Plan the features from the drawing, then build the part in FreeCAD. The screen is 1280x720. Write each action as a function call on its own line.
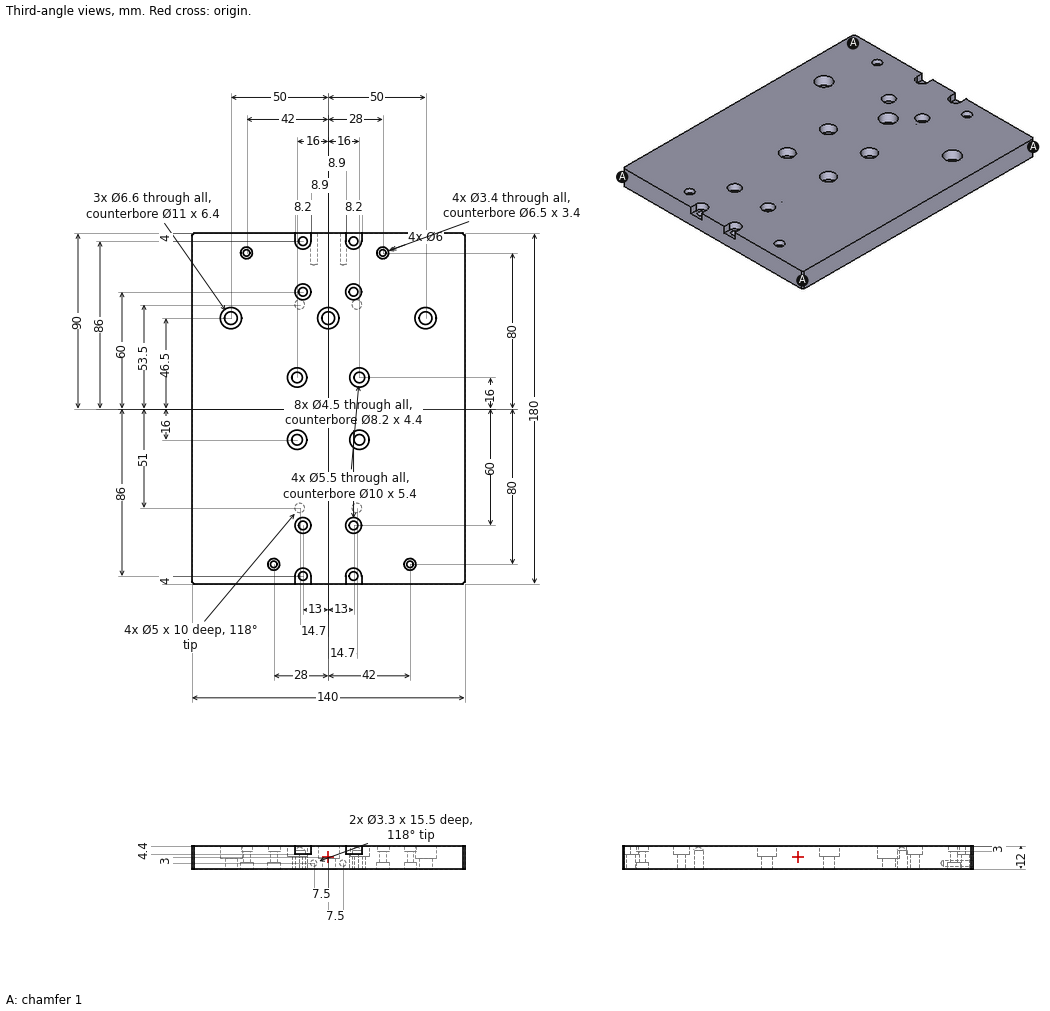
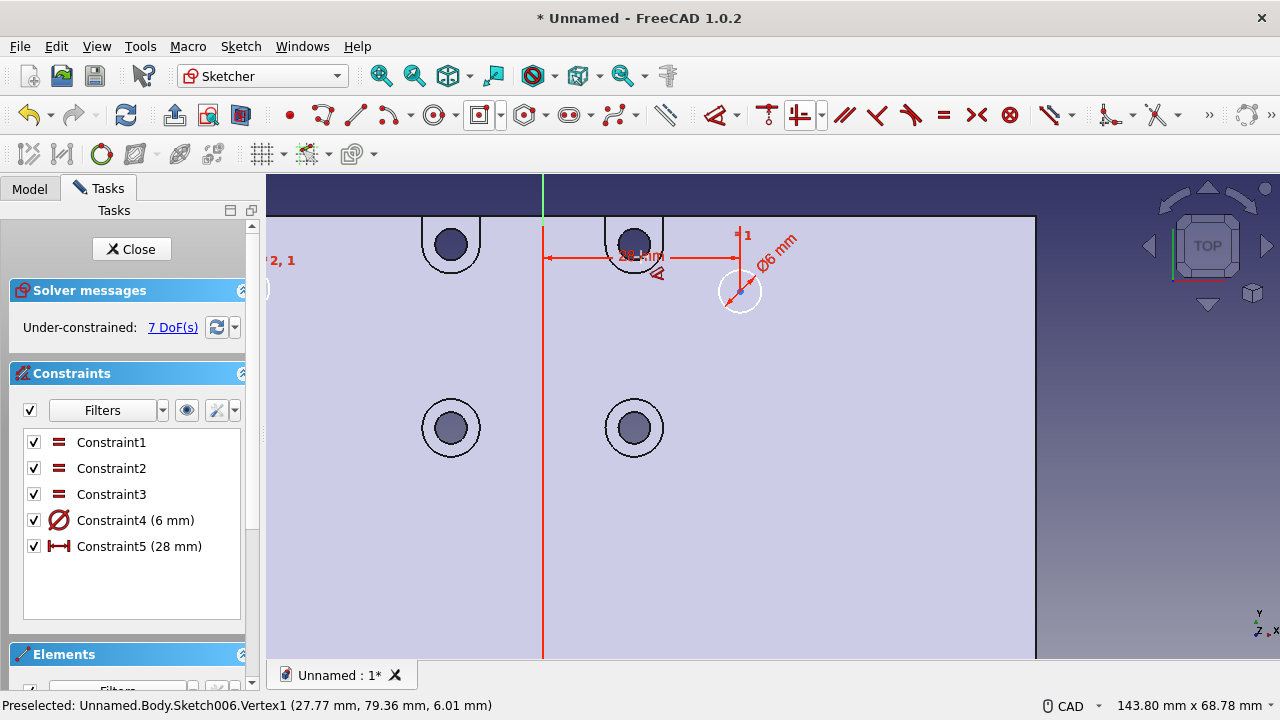
click(740, 291)
click(774, 461)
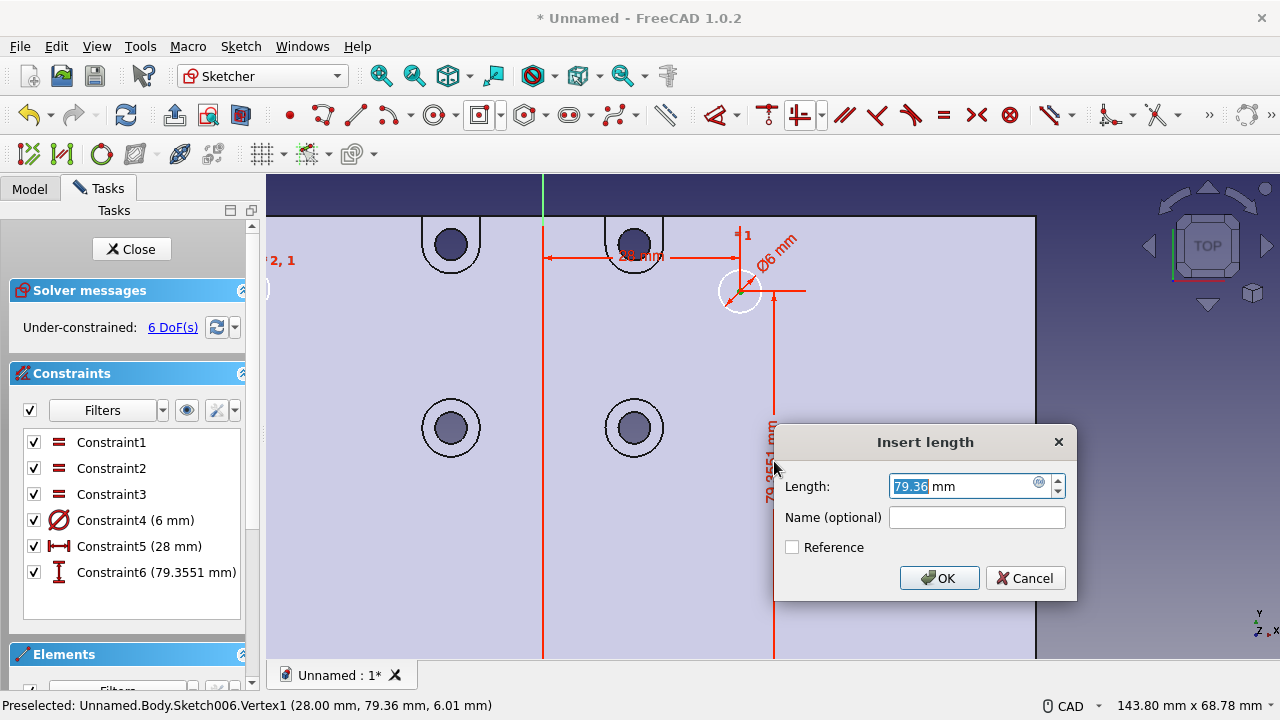
text(80)
key(Return)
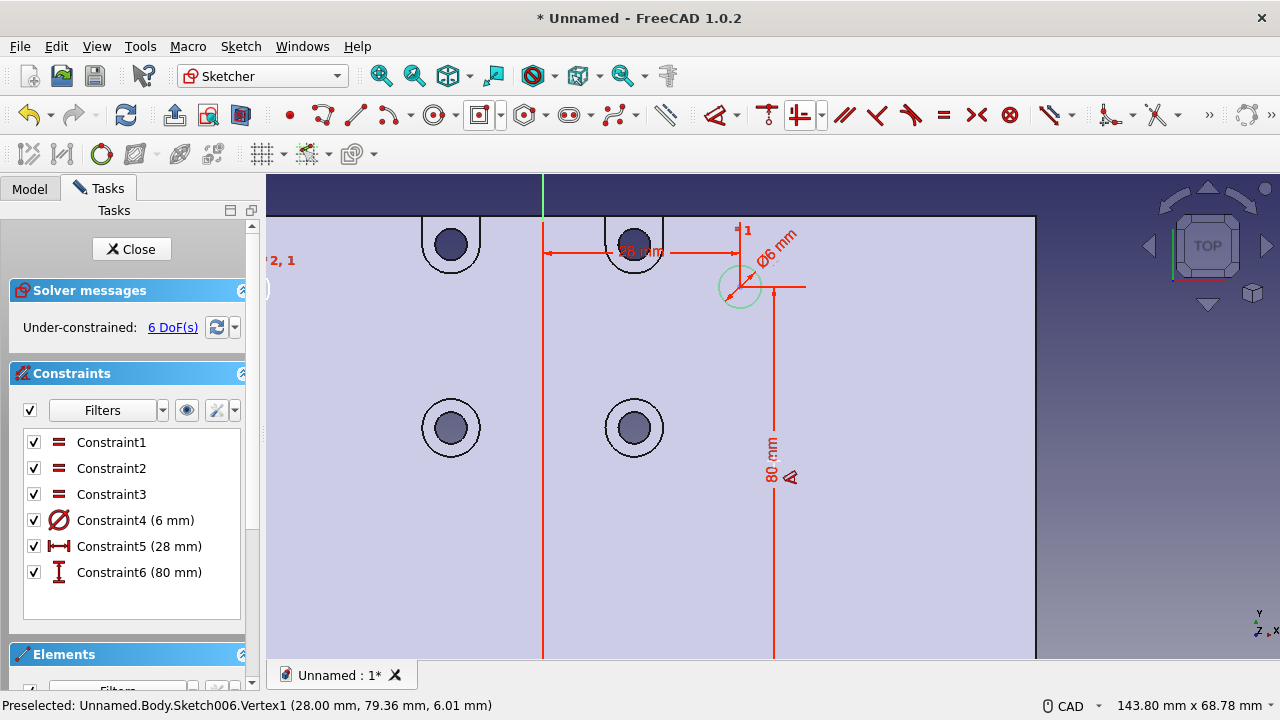
scroll(757, 274, down, 7)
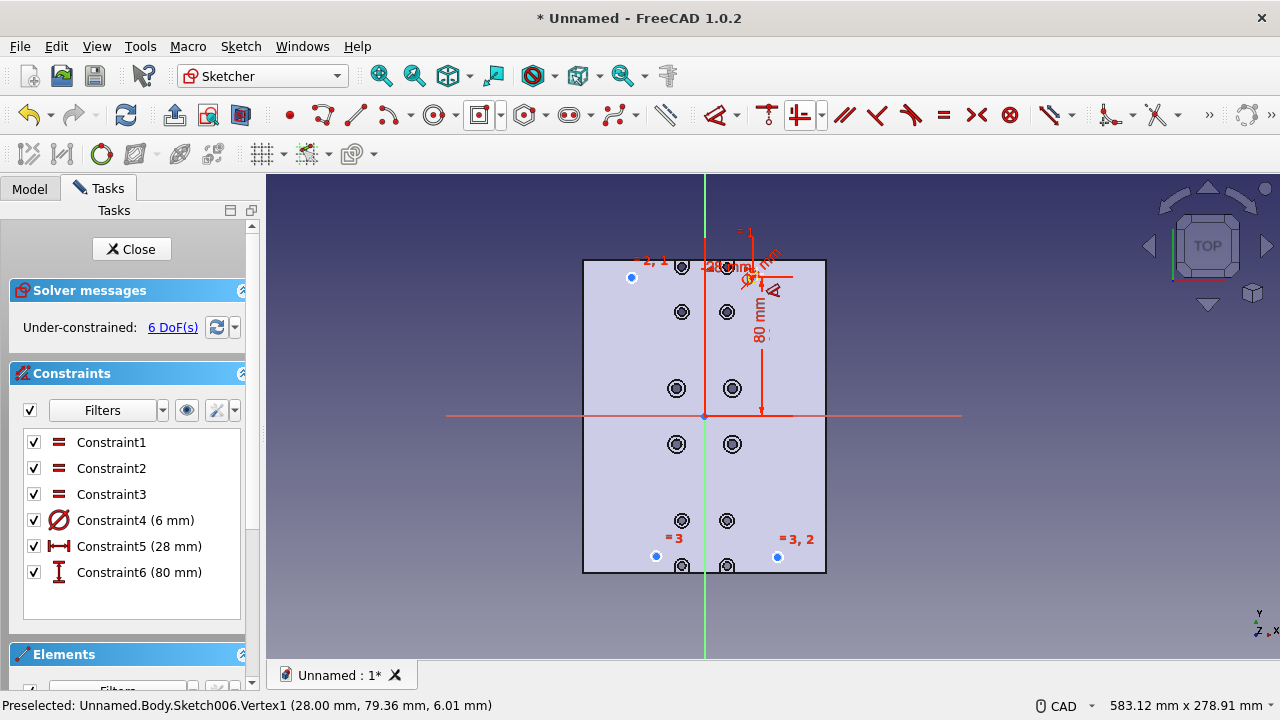
click(632, 278)
click(668, 244)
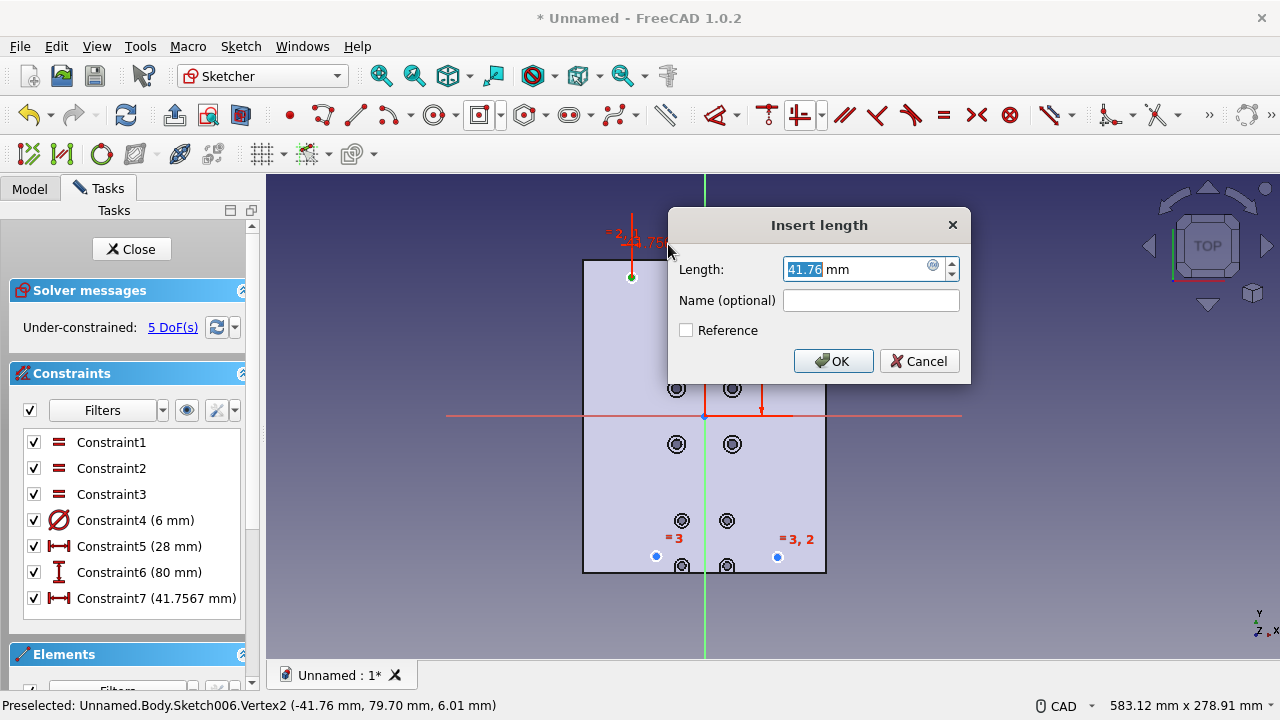
text(42)
key(Return)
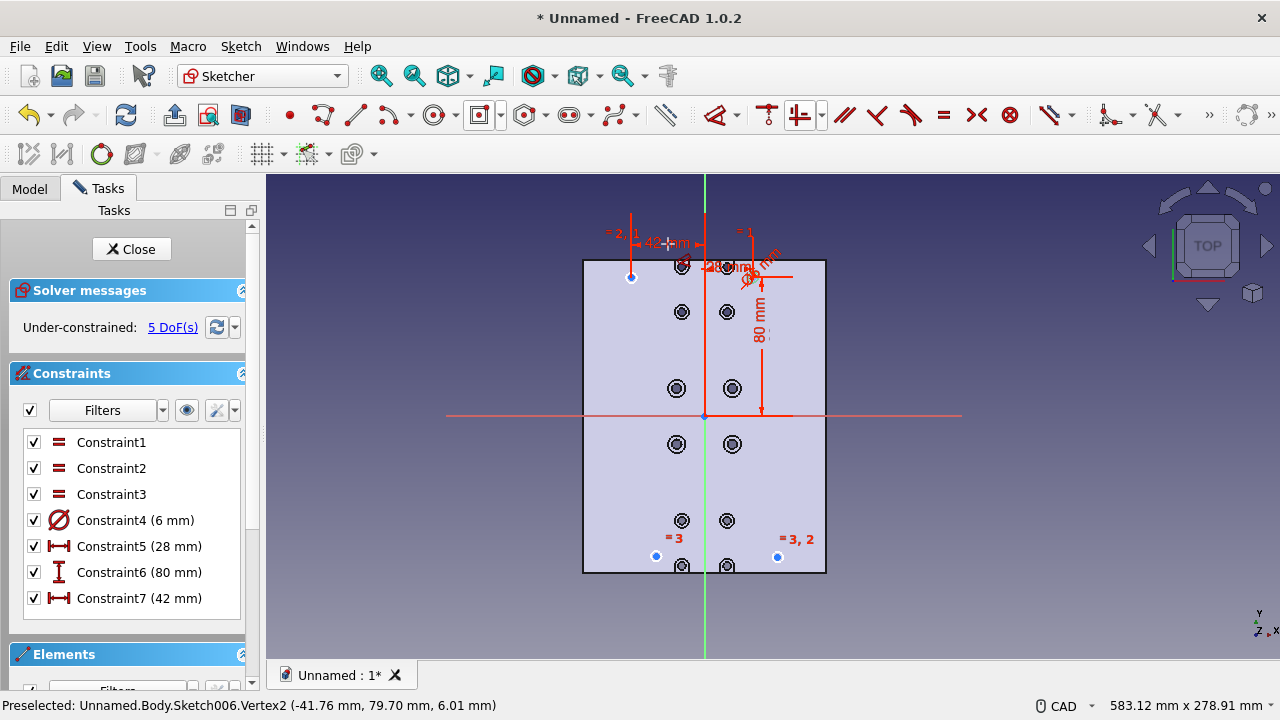
click(631, 278)
click(597, 347)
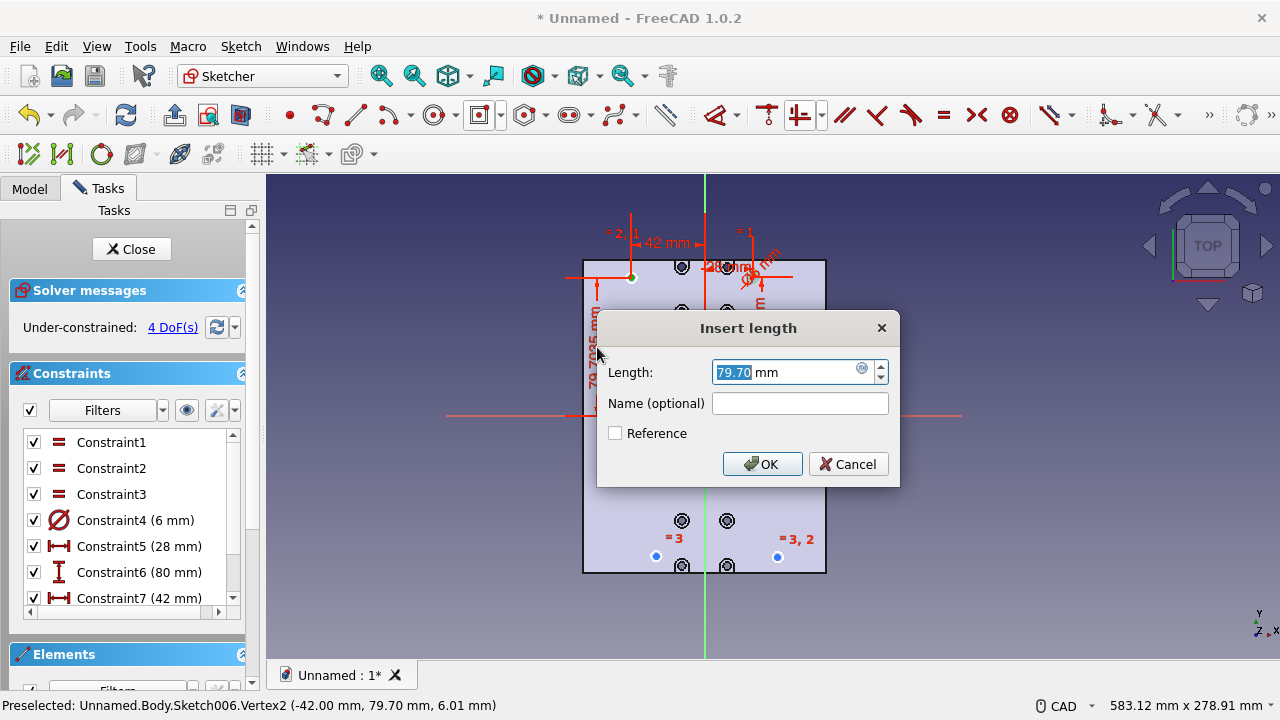
text(80)
key(Return)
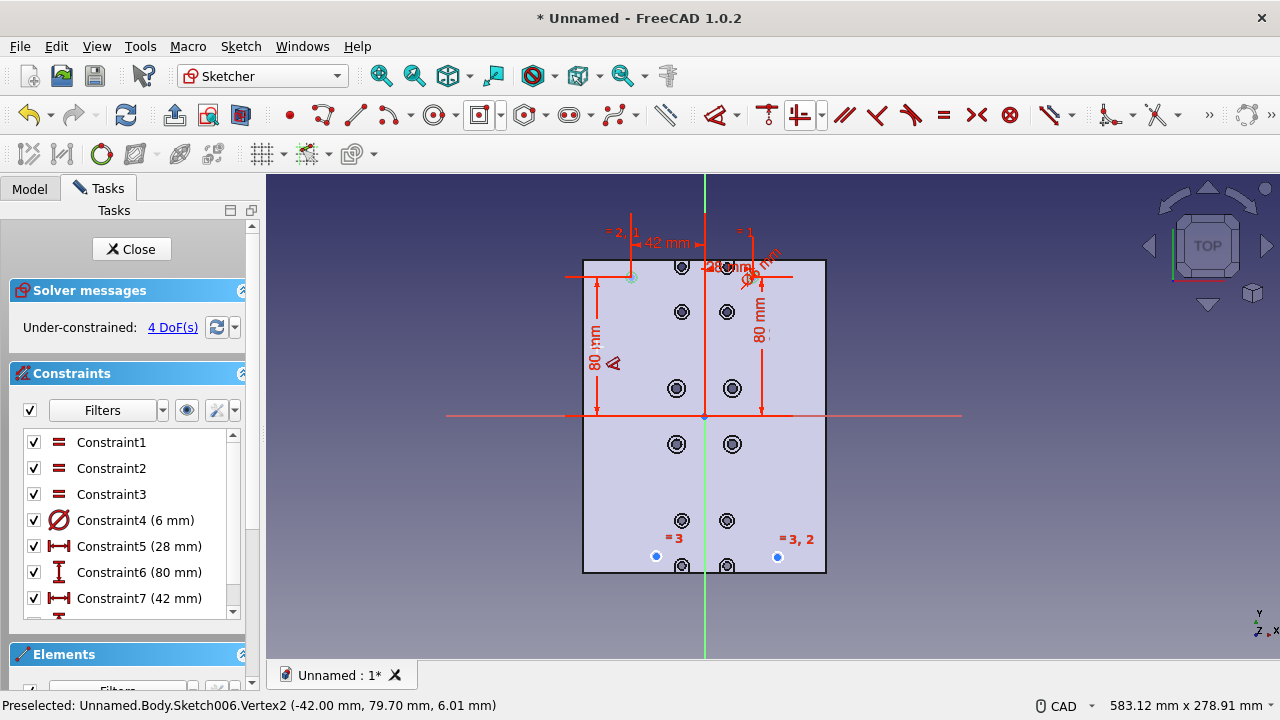
click(778, 557)
click(741, 591)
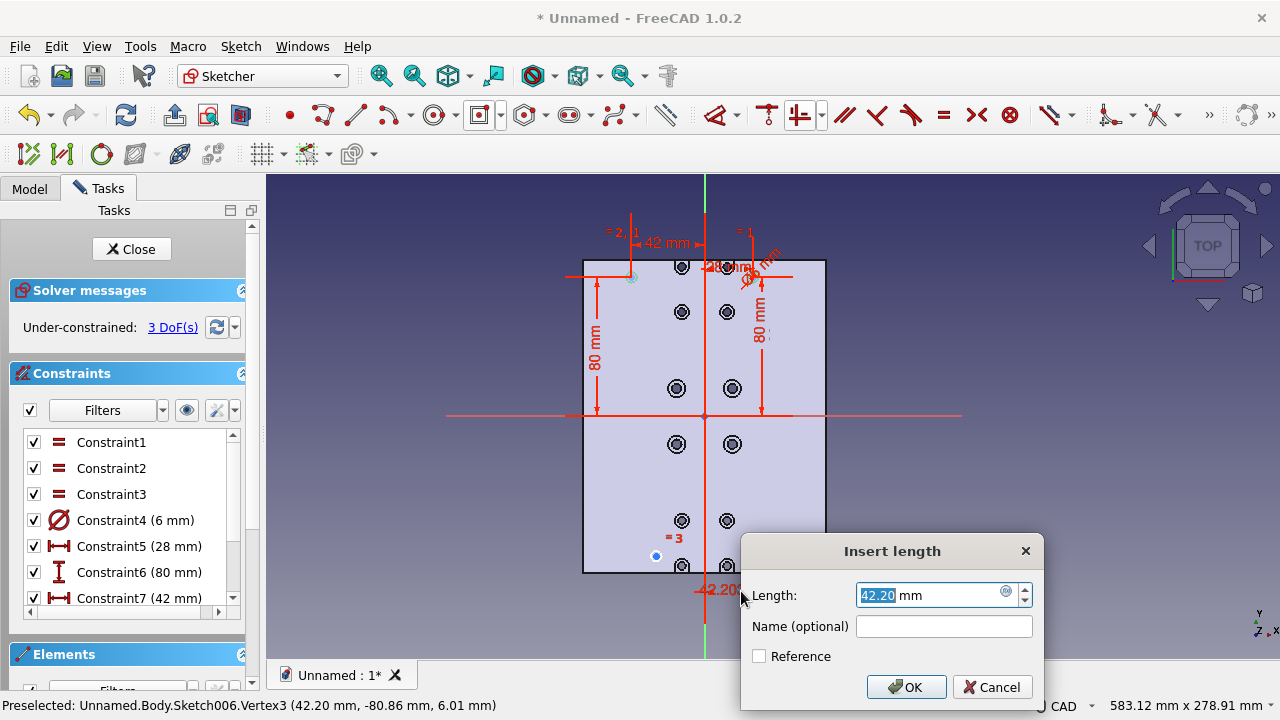
text(42)
key(Return)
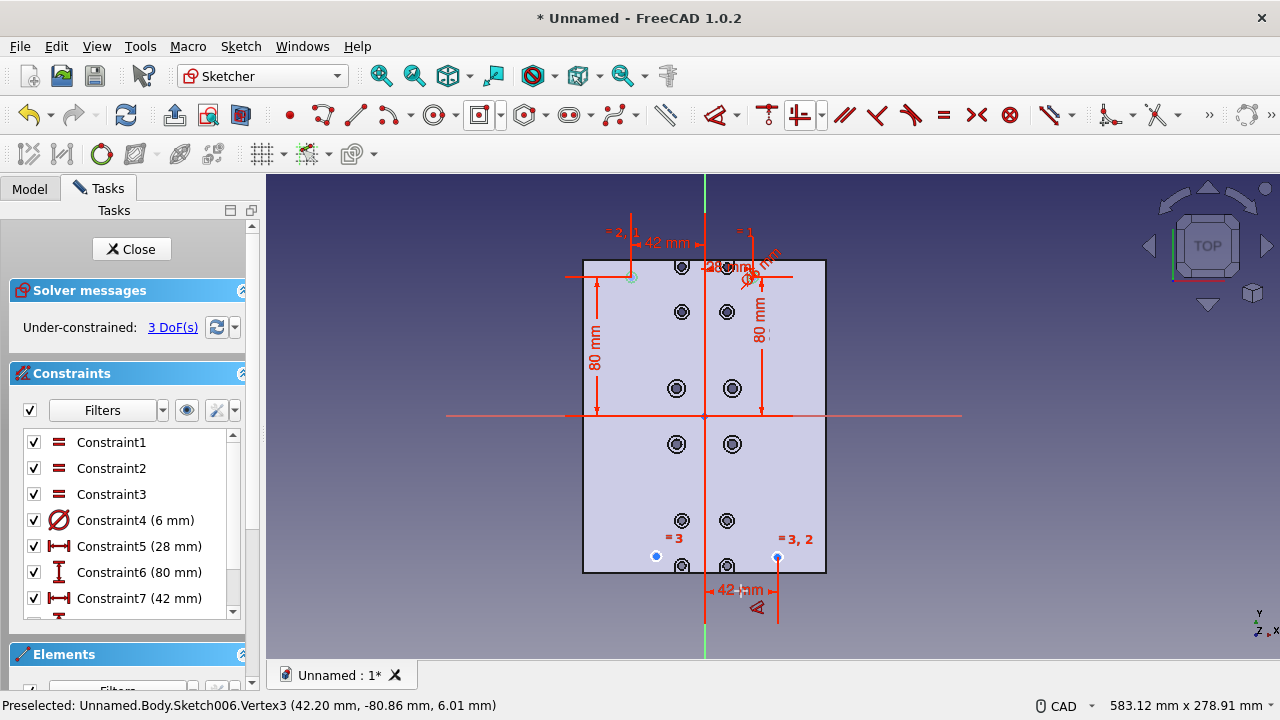
click(778, 557)
click(812, 487)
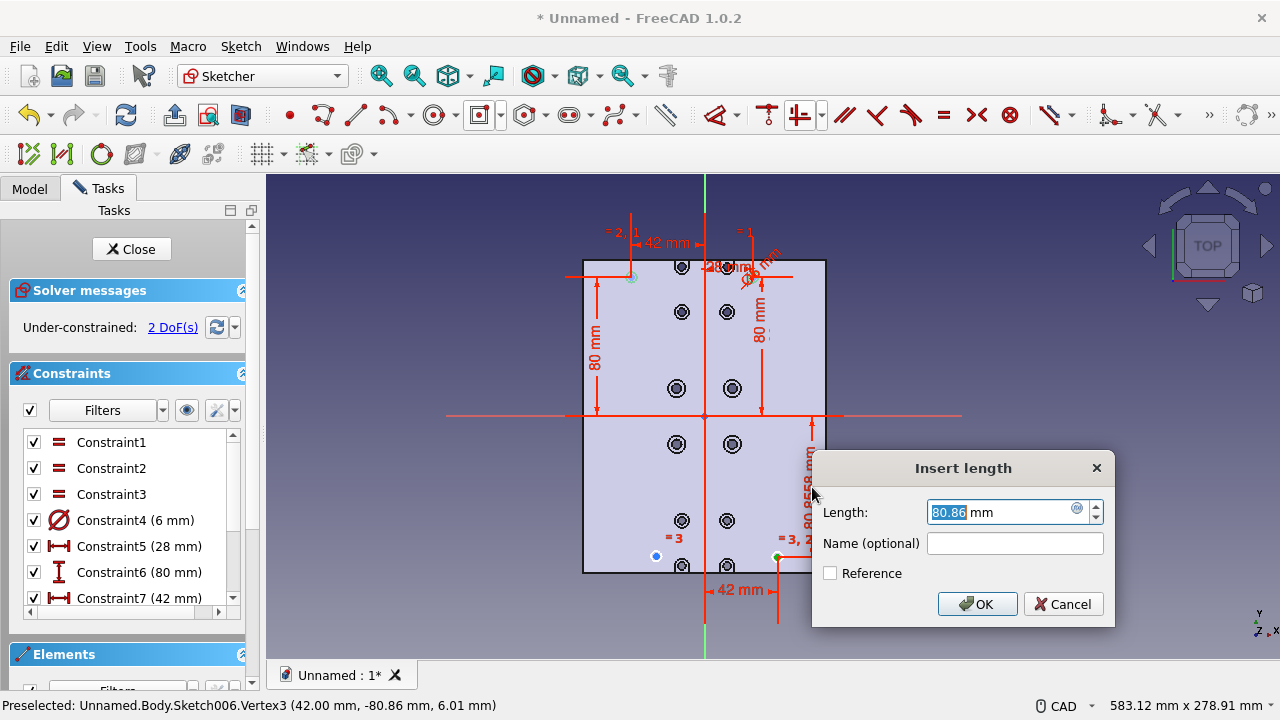
text(80)
key(Return)